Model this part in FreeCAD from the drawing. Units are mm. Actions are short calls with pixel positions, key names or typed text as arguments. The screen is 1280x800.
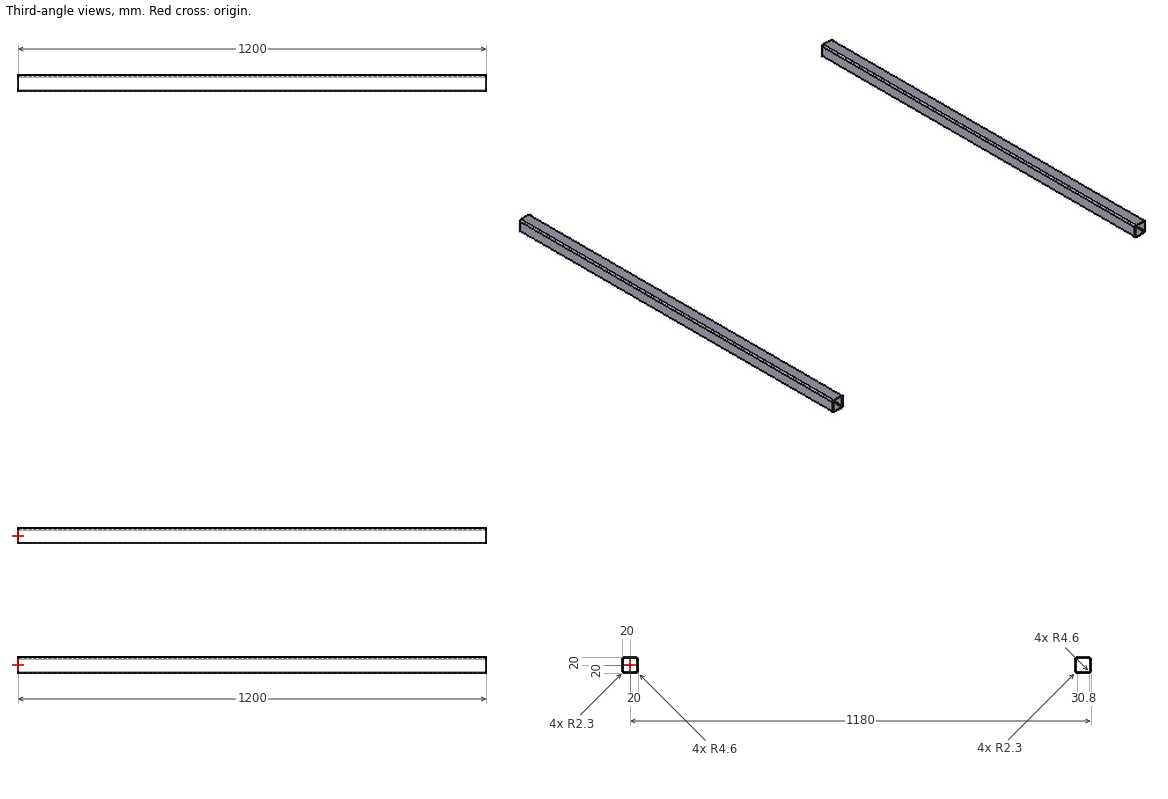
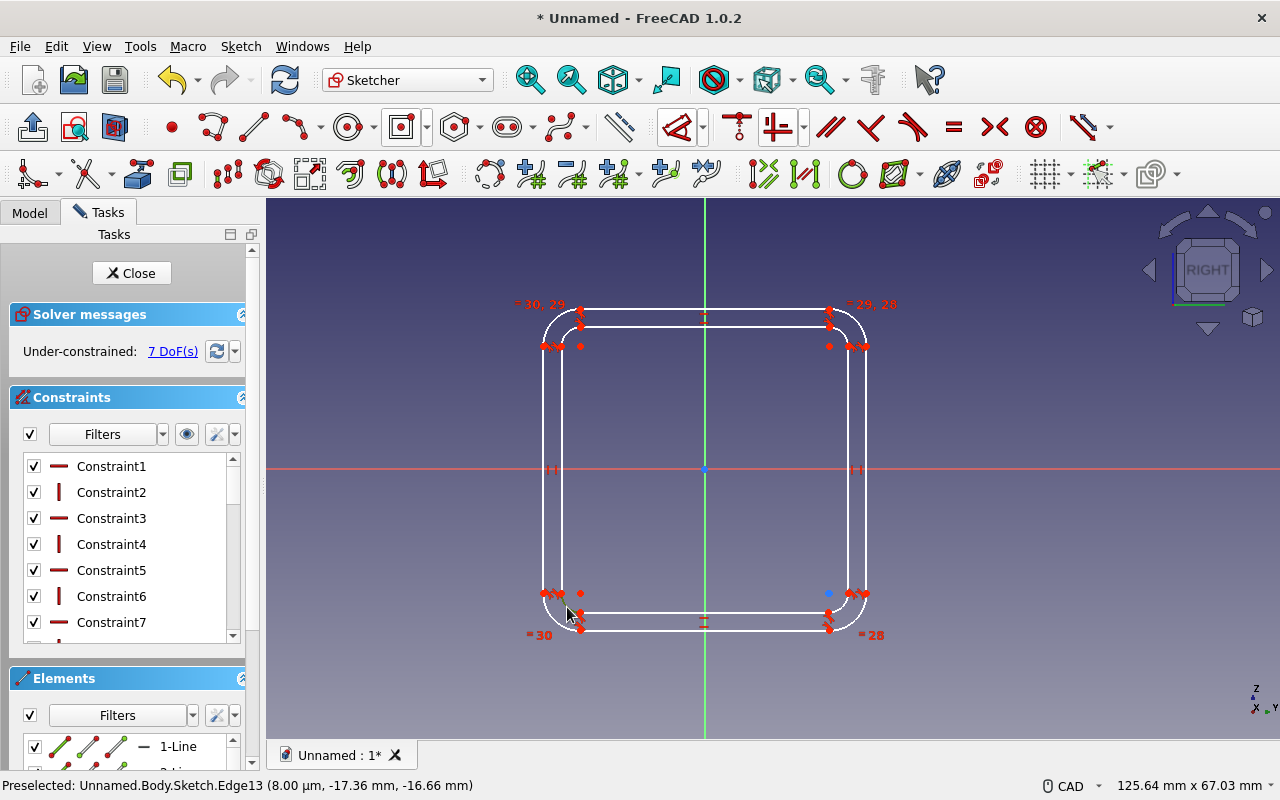
click(842, 607)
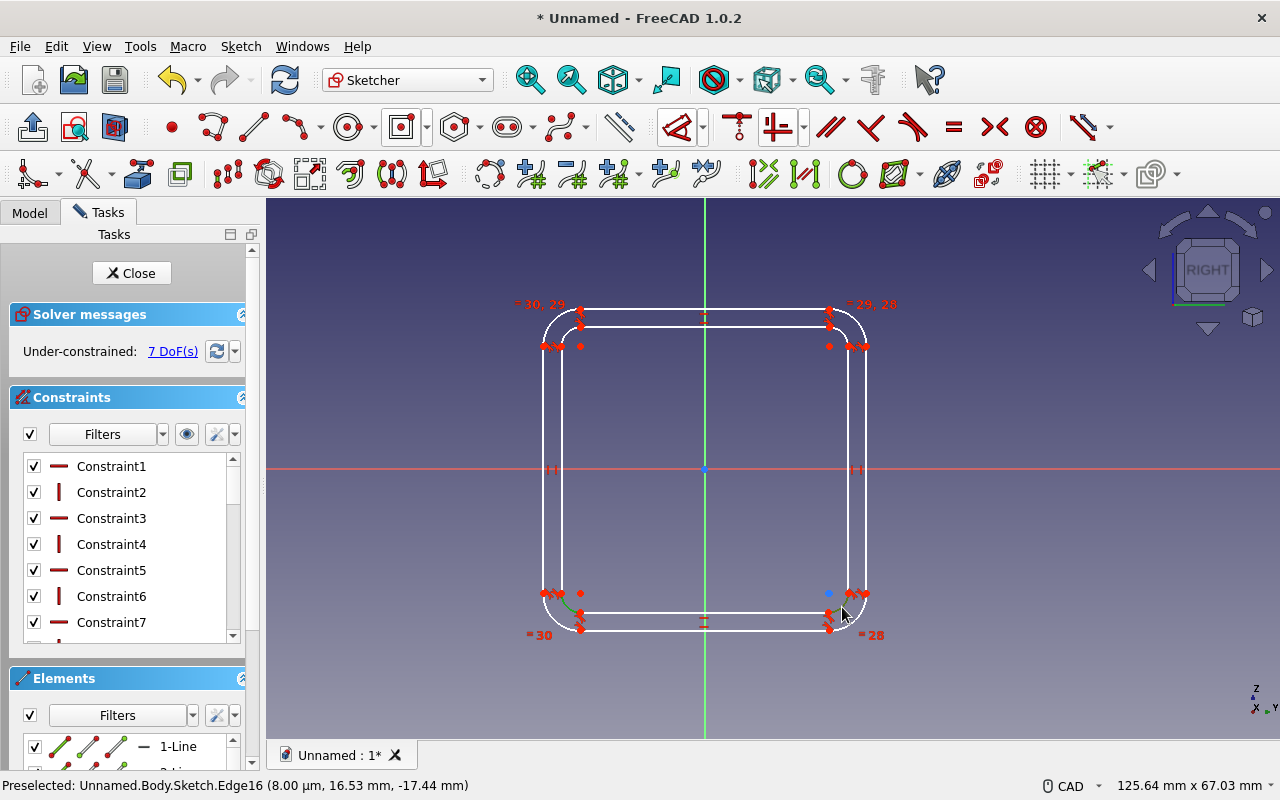
key(e)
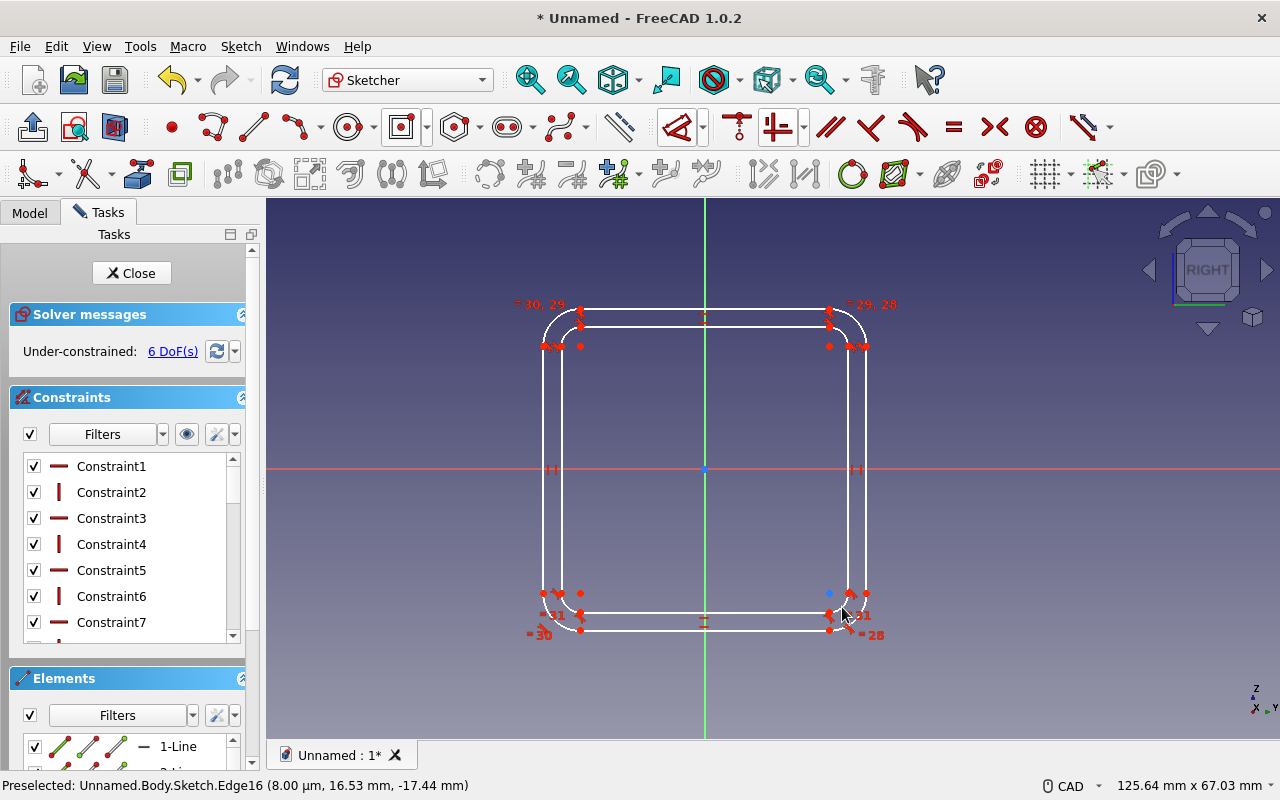
click(841, 629)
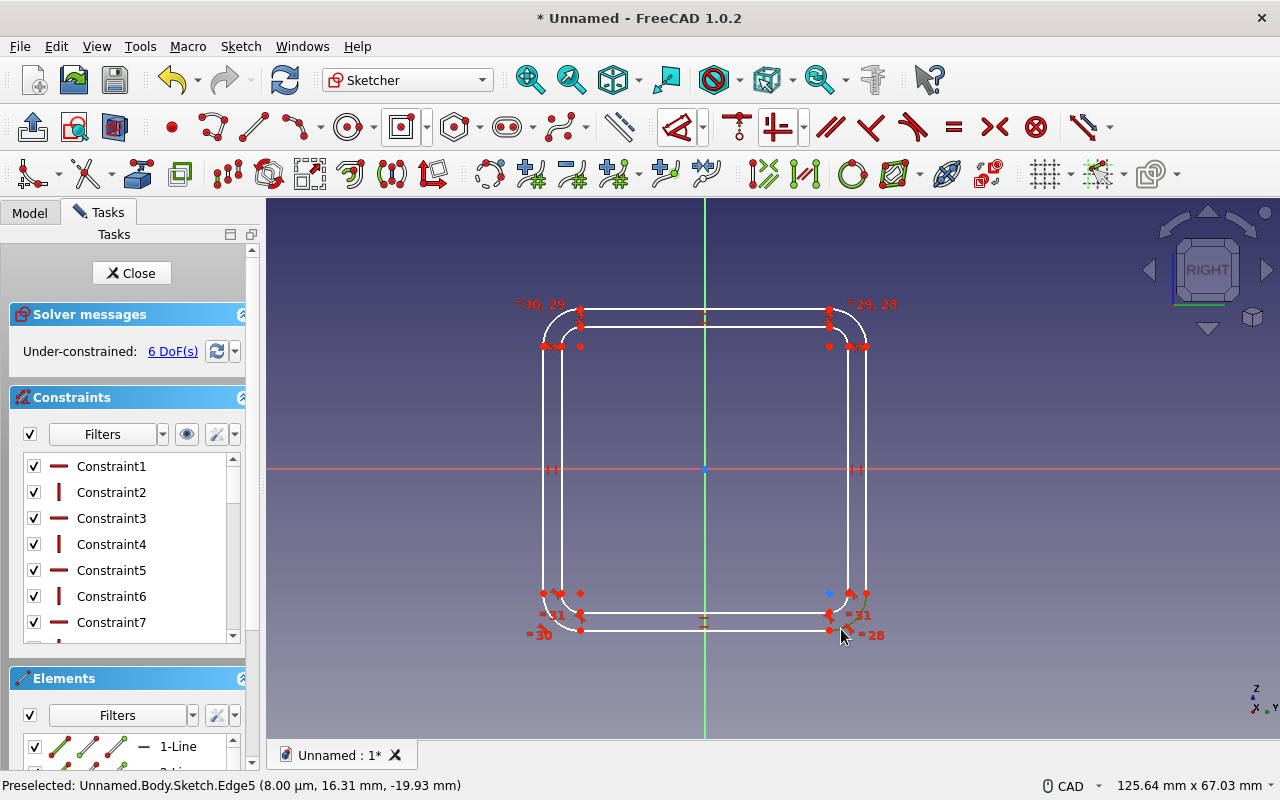
key(k)
key(r)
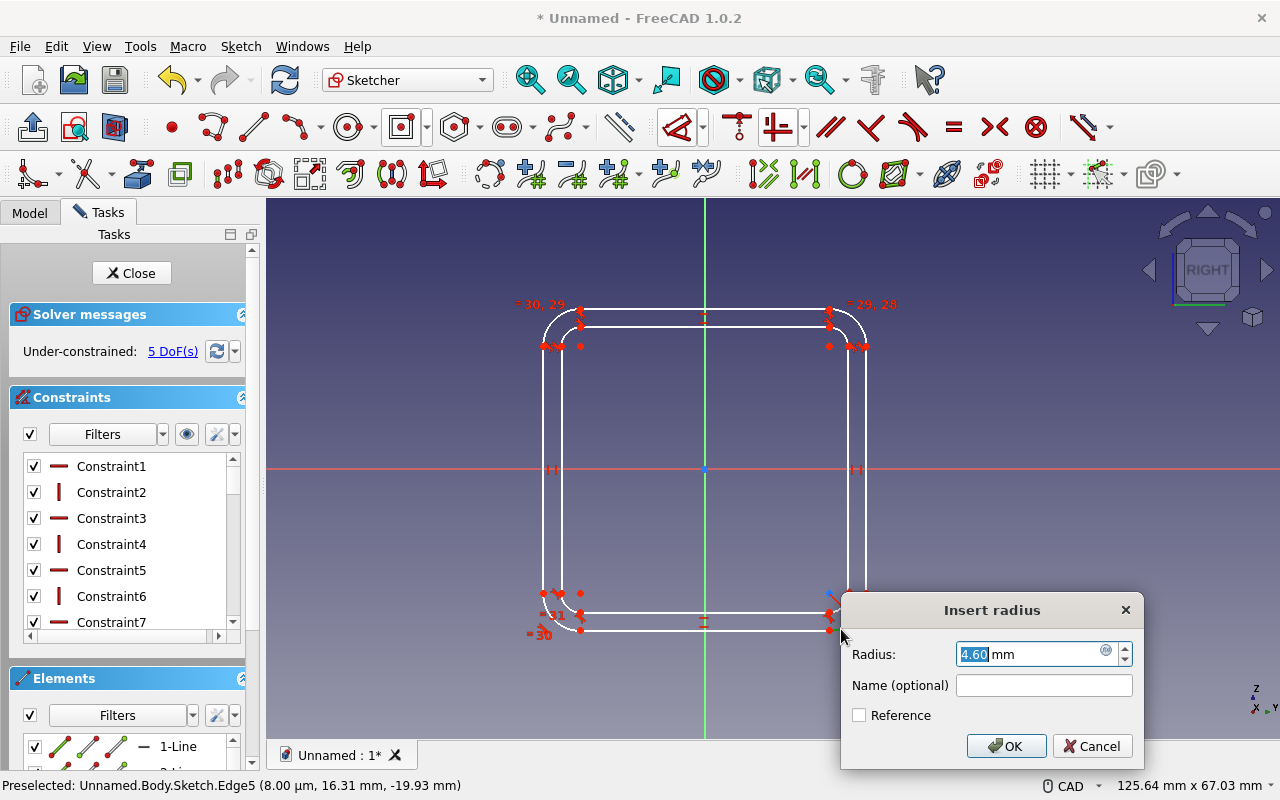
text(4.6)
key(Return)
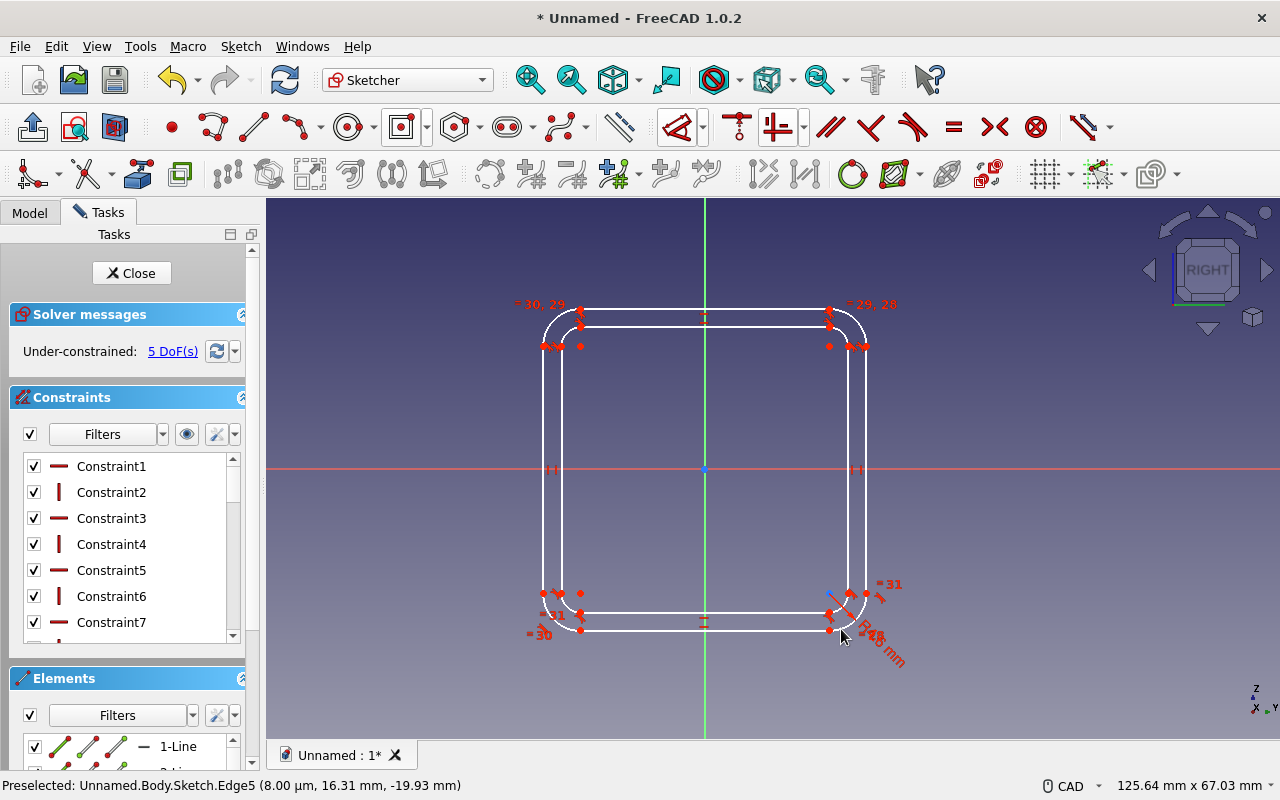
scroll(567, 607, up, 4)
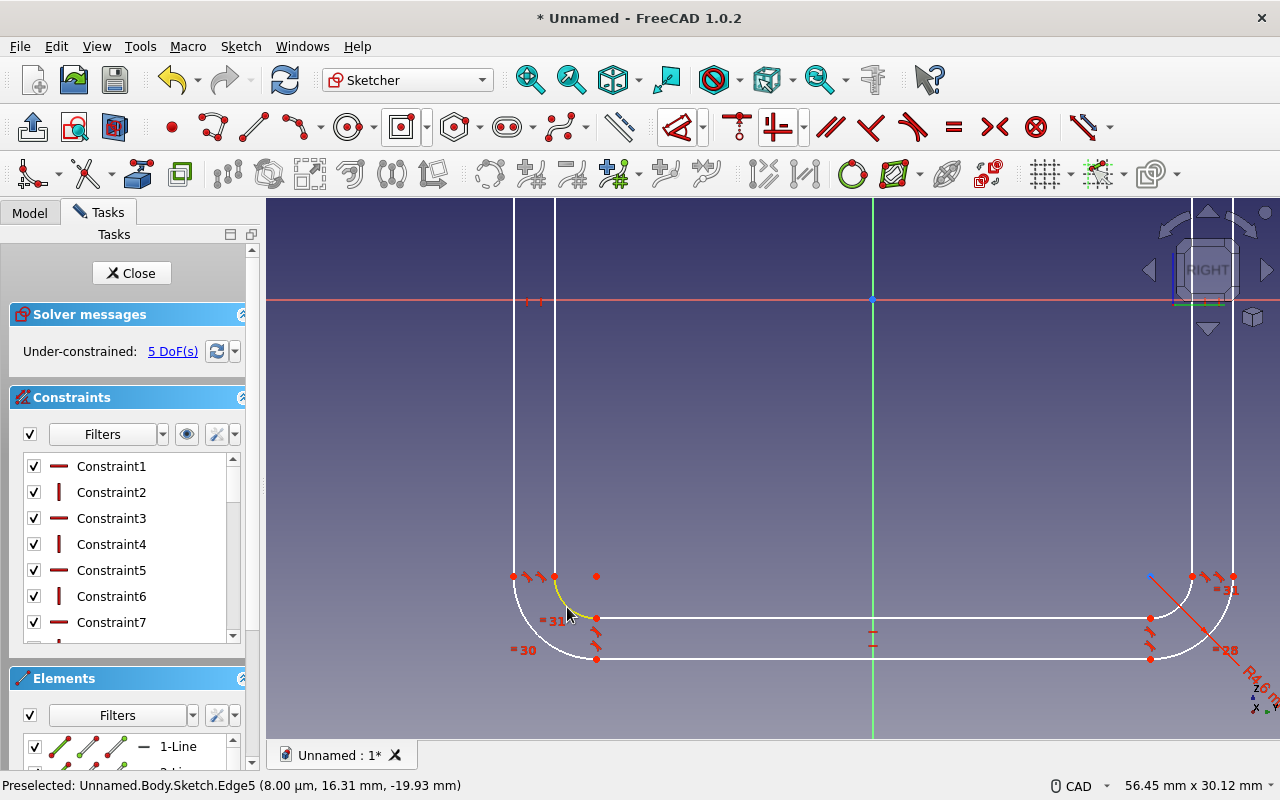
click(567, 606)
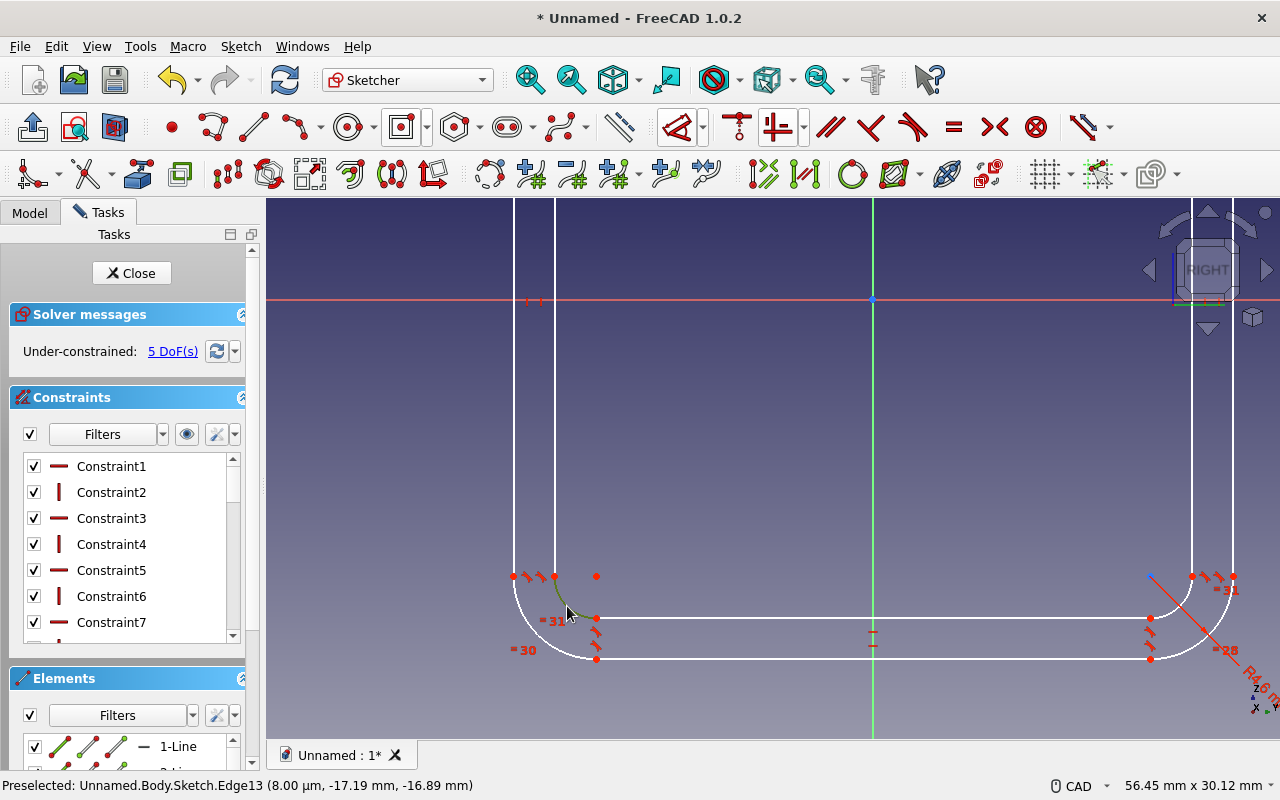
key(k)
key(r)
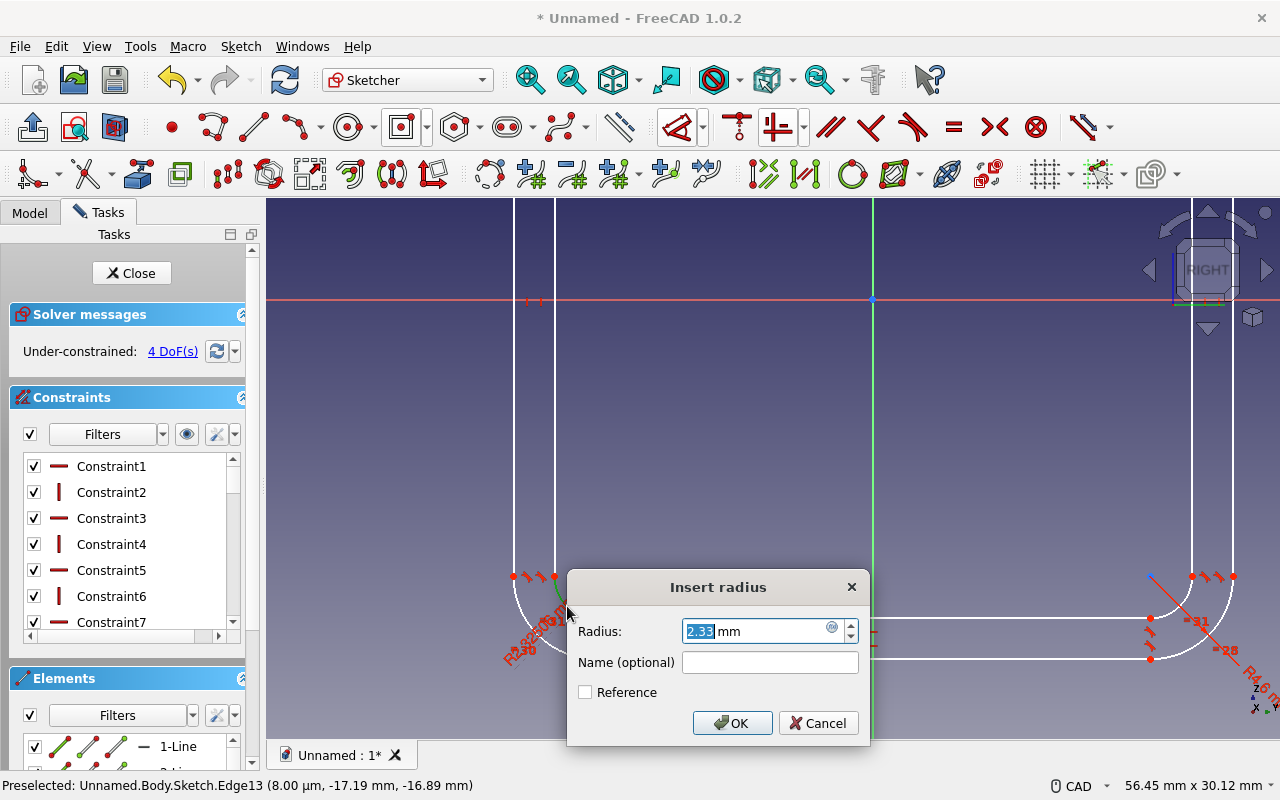
text(2.3)
key(Return)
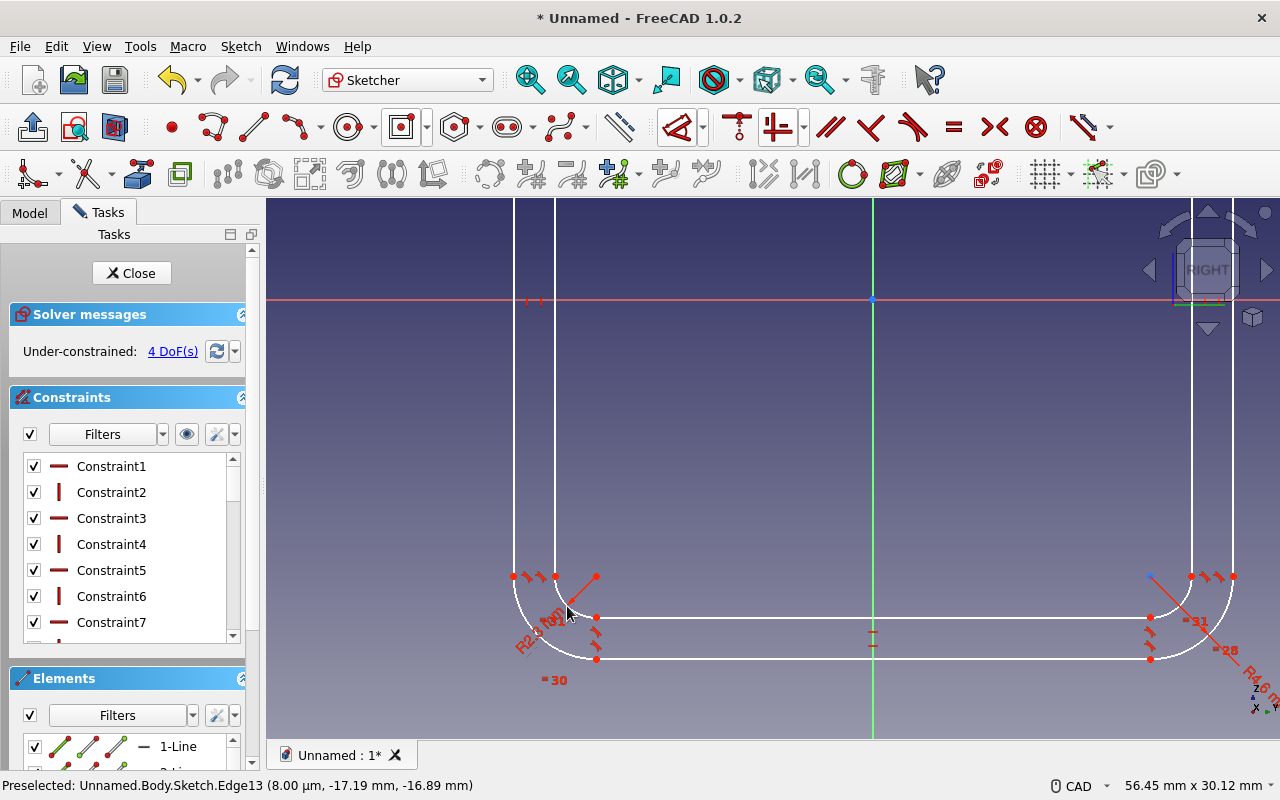
click(596, 659)